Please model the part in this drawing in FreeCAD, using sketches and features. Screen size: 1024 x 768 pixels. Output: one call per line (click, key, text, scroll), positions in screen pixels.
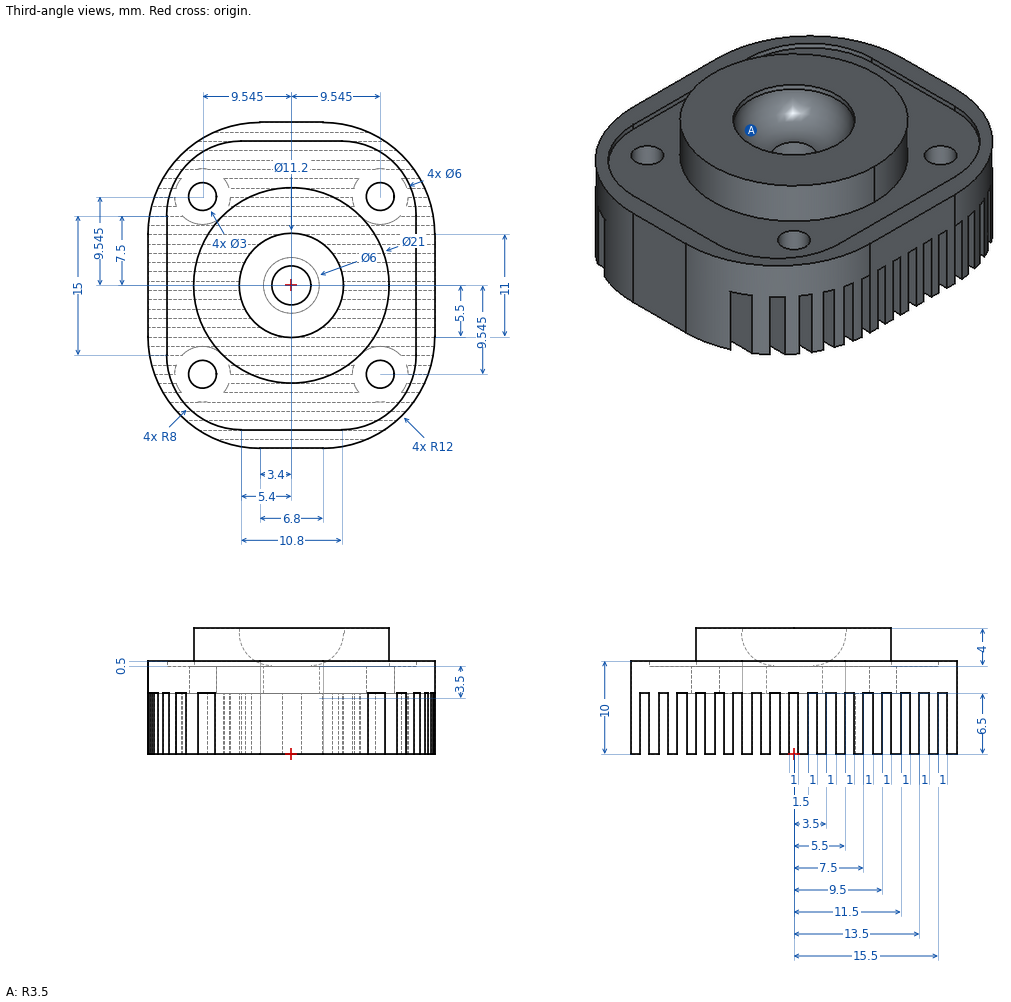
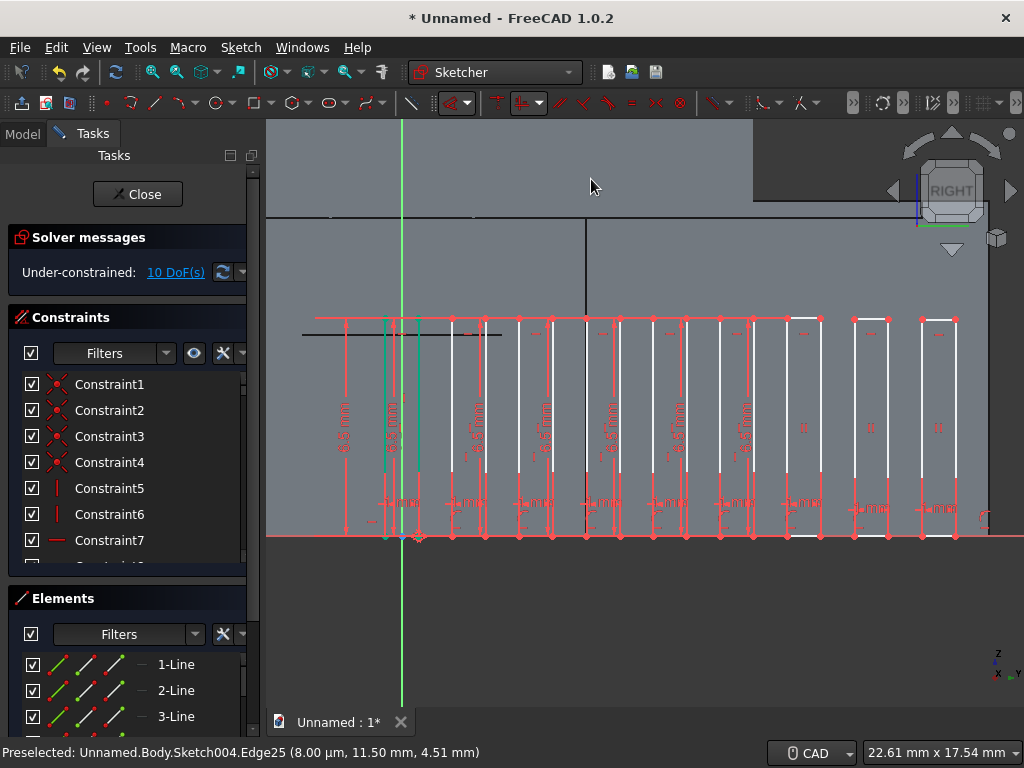
click(855, 384)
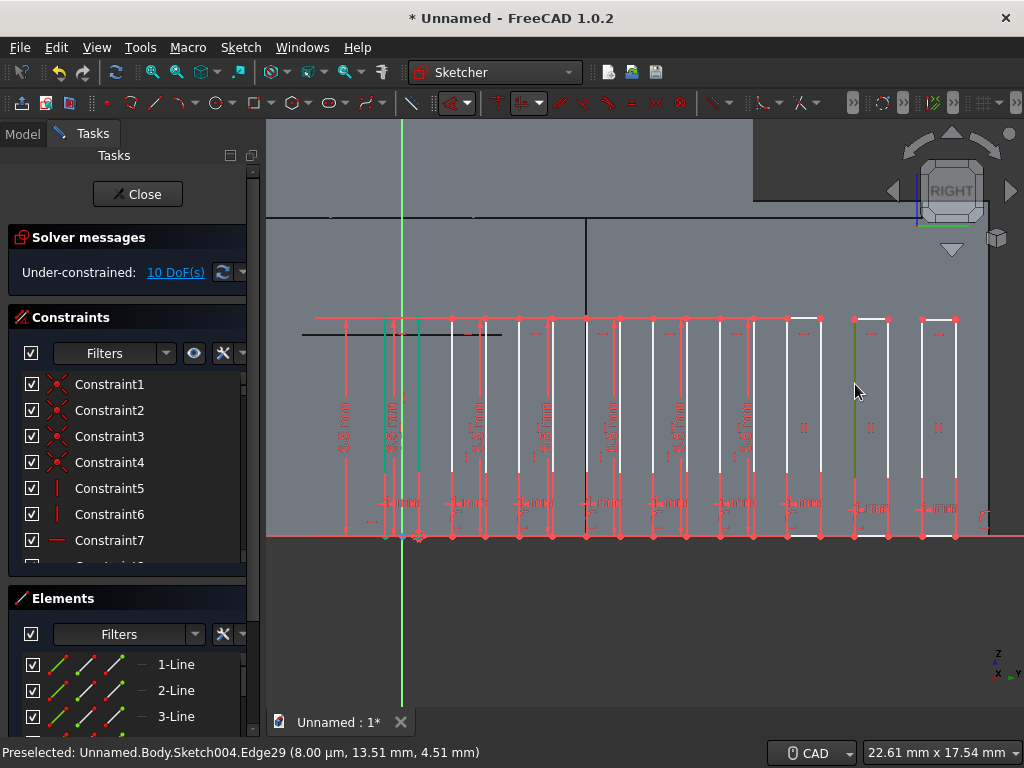
key(i)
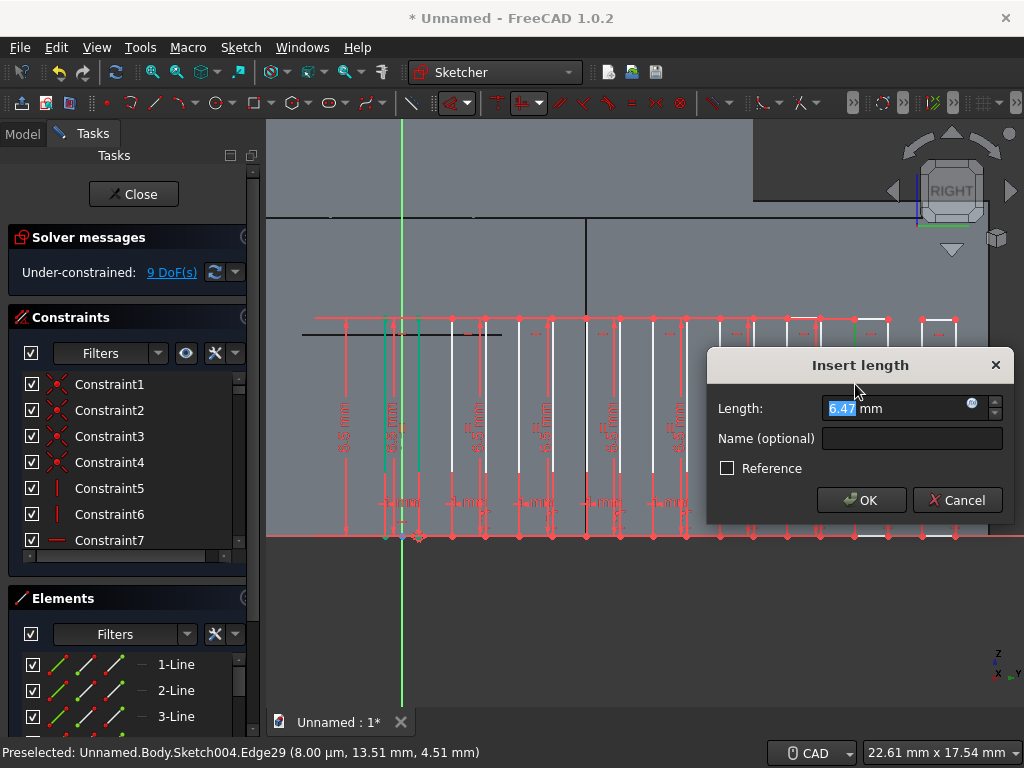
text(6.5)
key(Return)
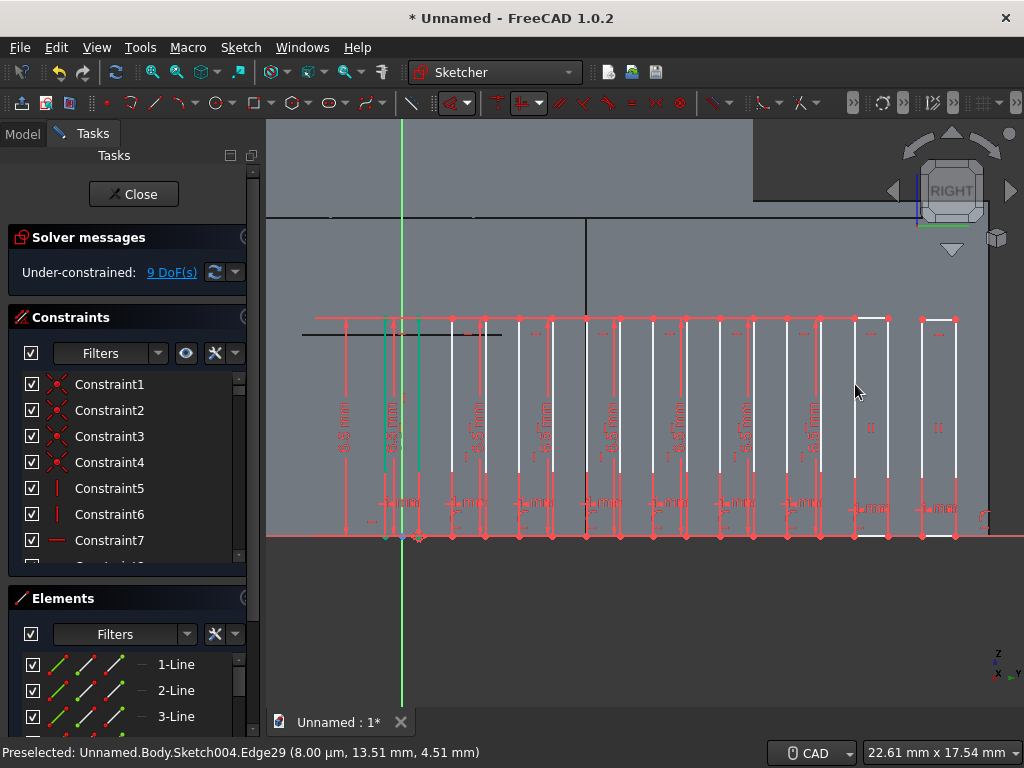
scroll(386, 384, down, 2)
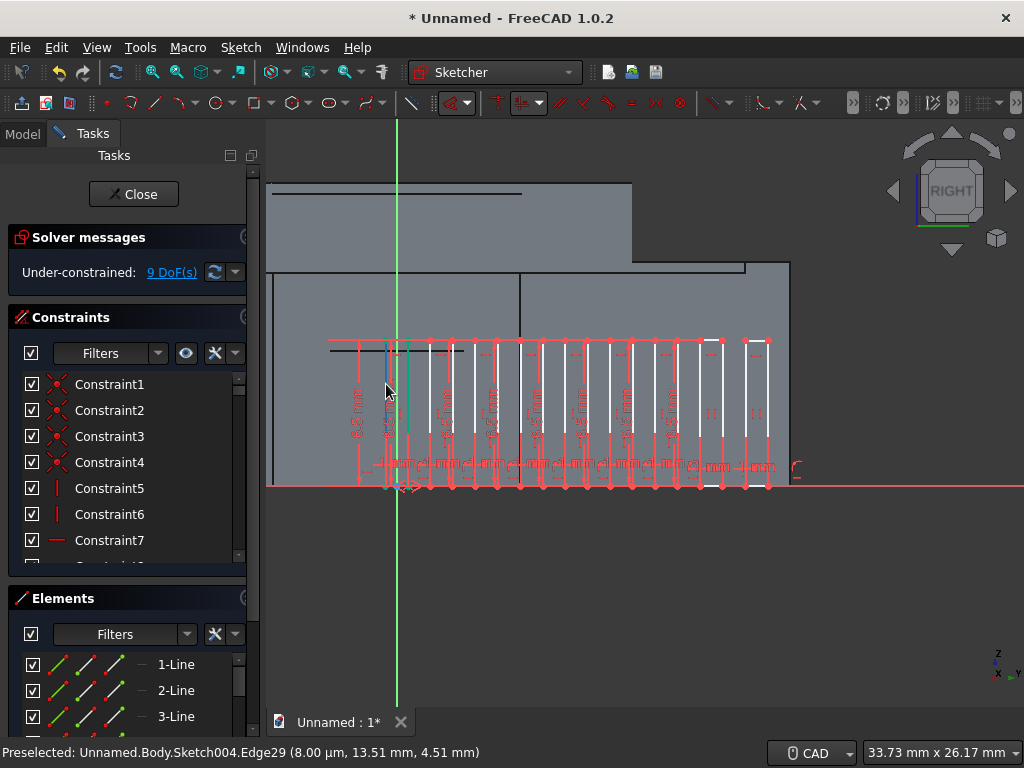
click(746, 385)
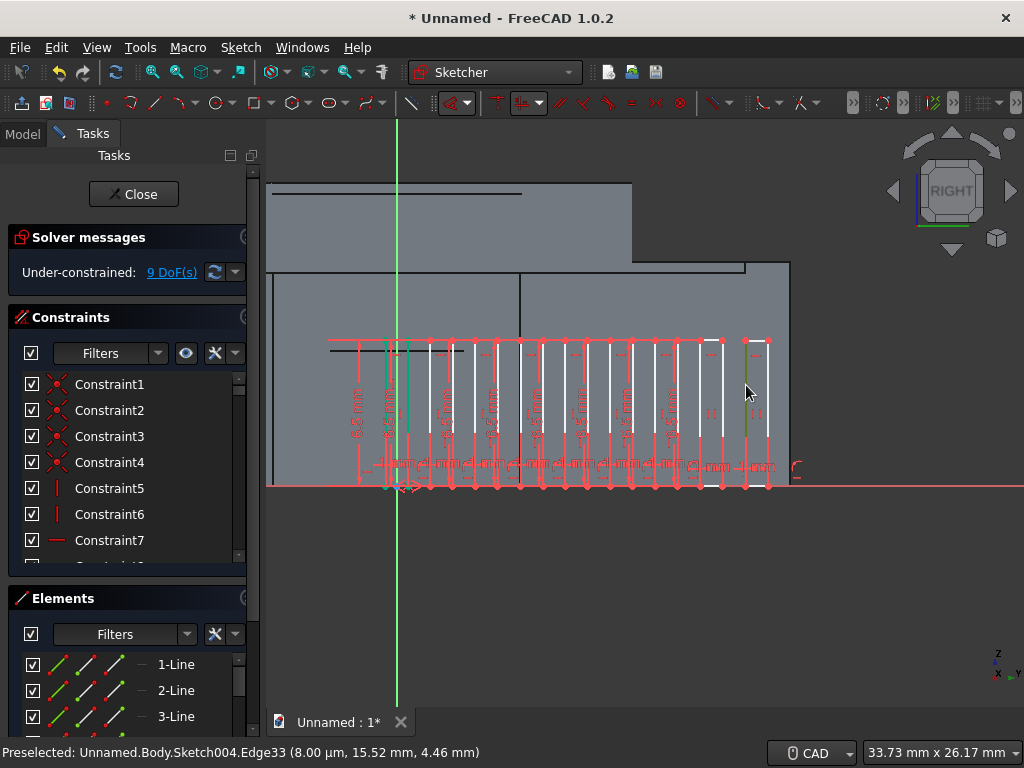
click(470, 104)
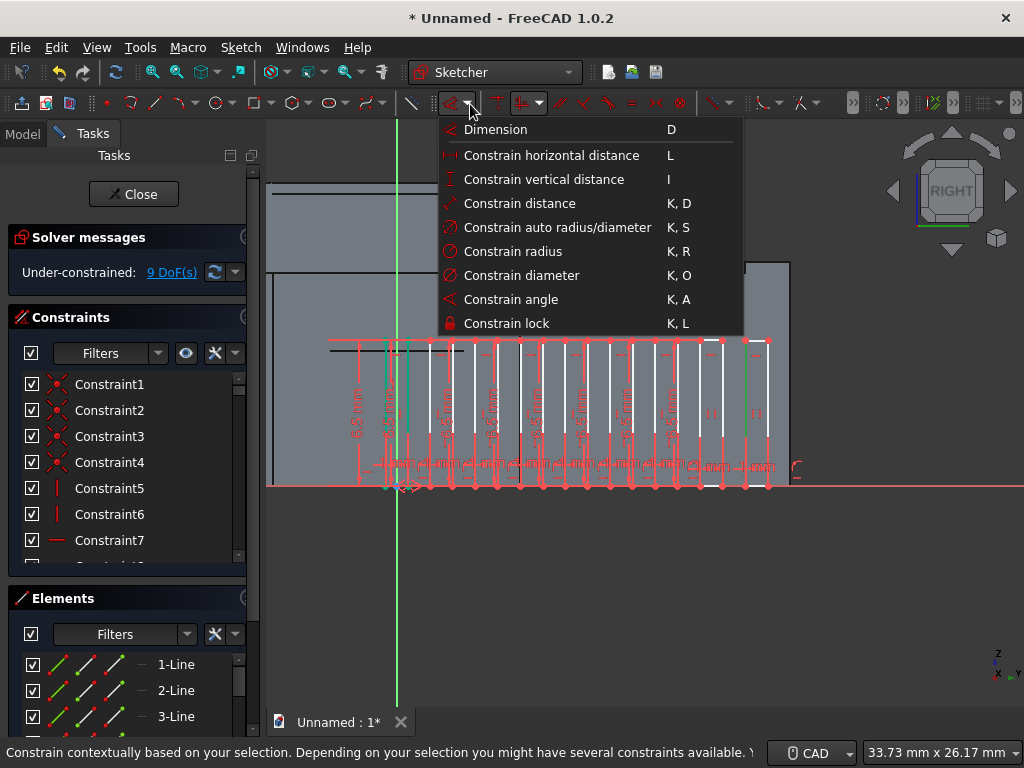
click(591, 179)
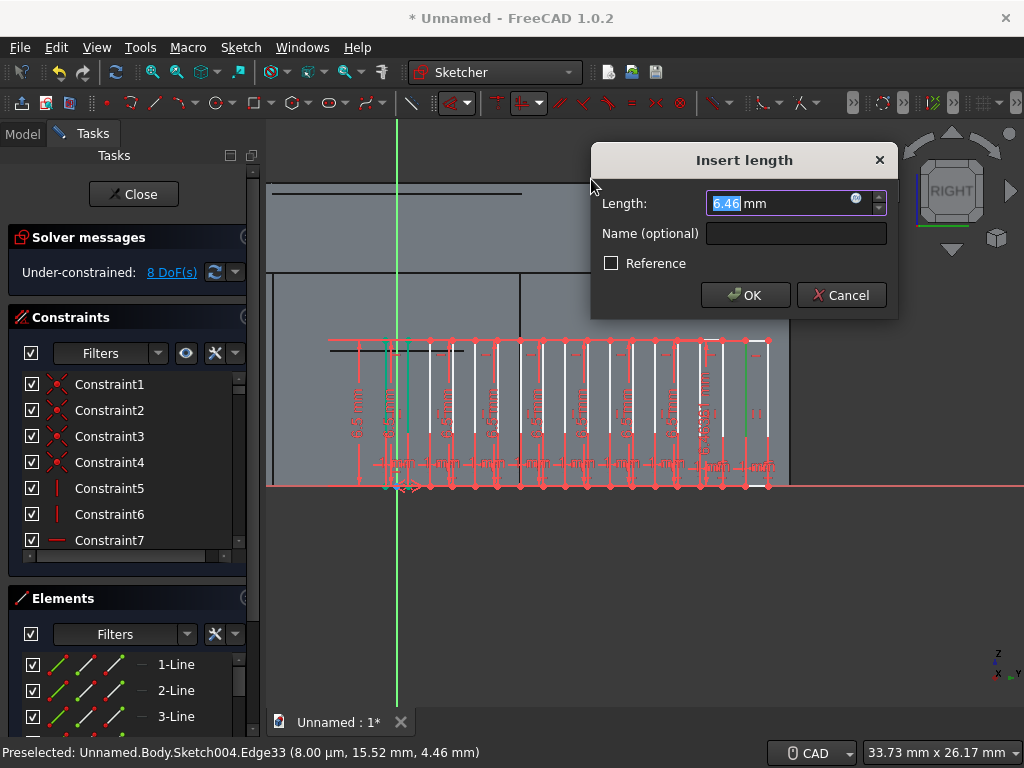
text(6.5)
key(Return)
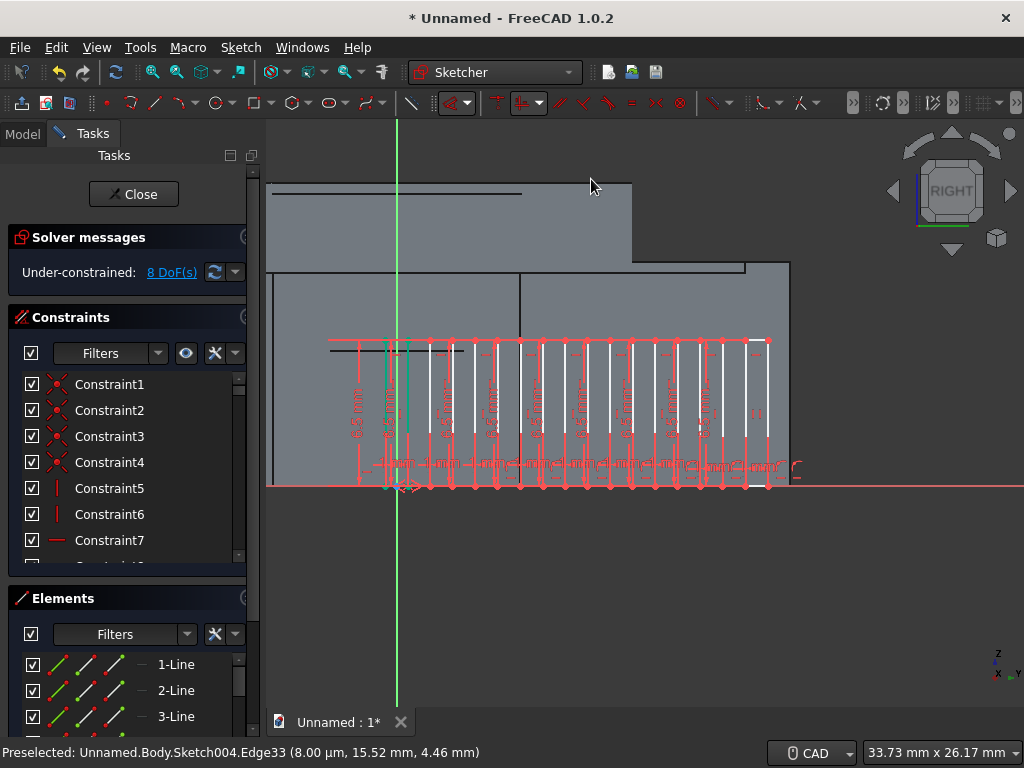
click(430, 340)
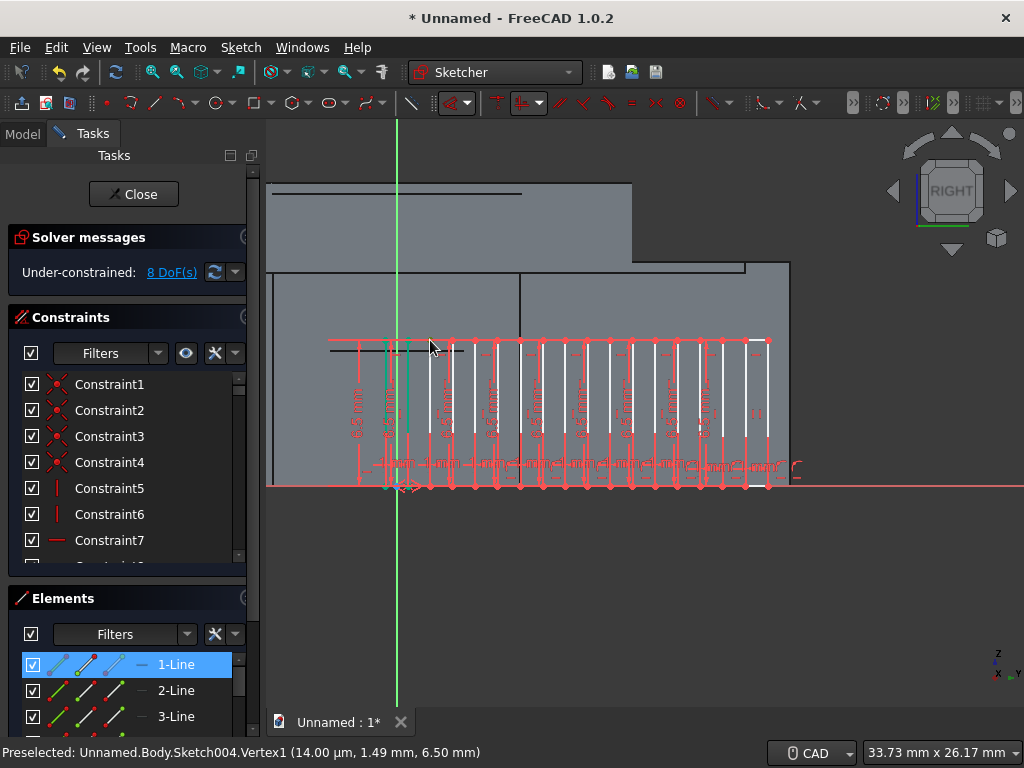
key(l)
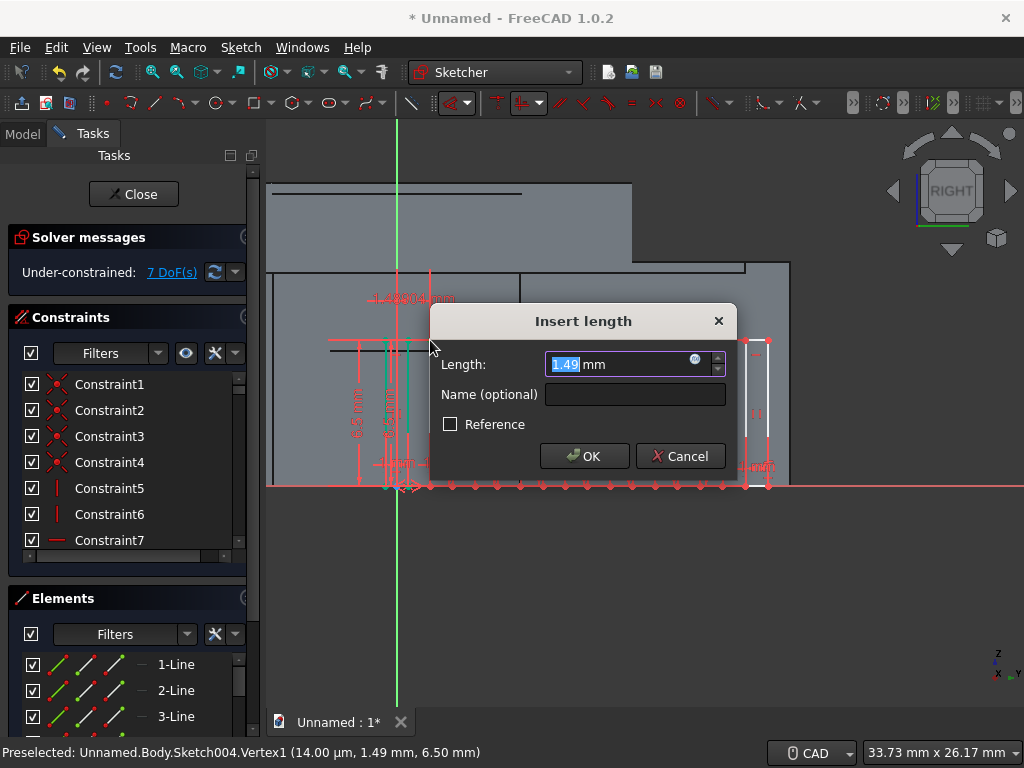
text(1.5)
key(Return)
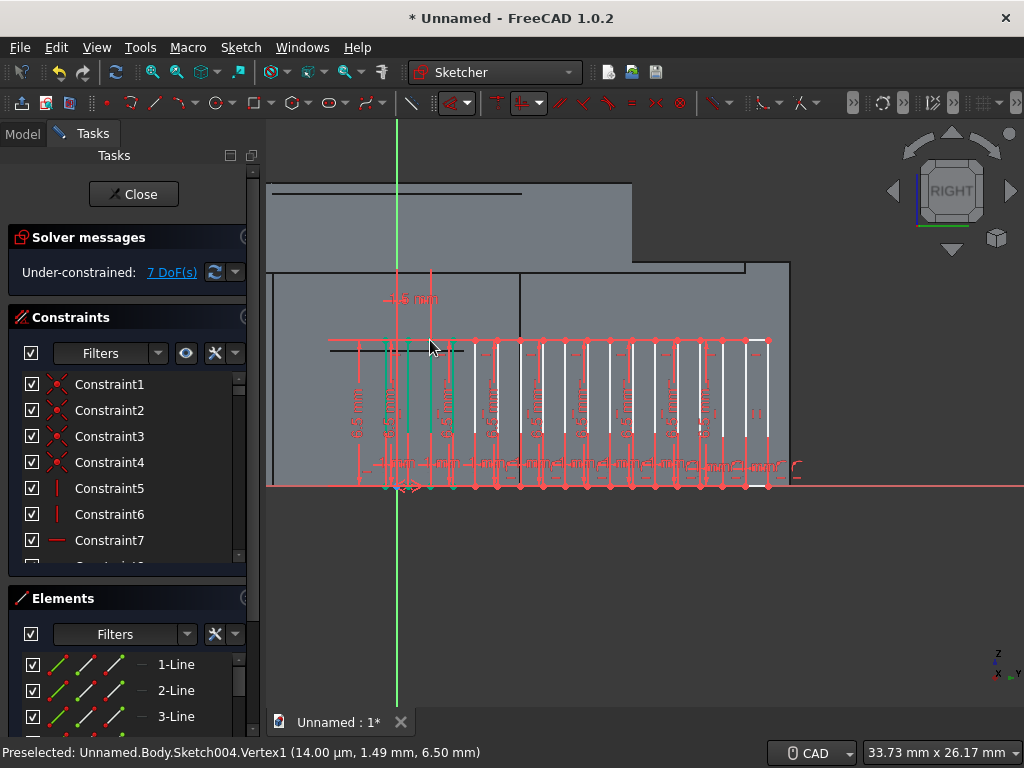
click(475, 340)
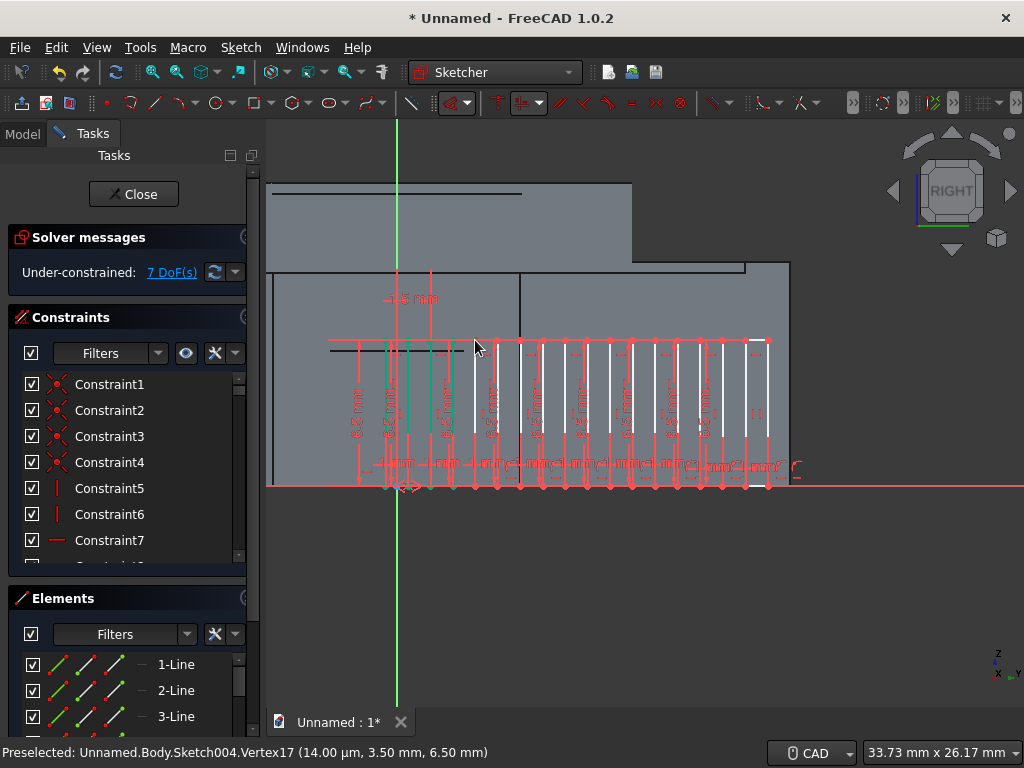
key(l)